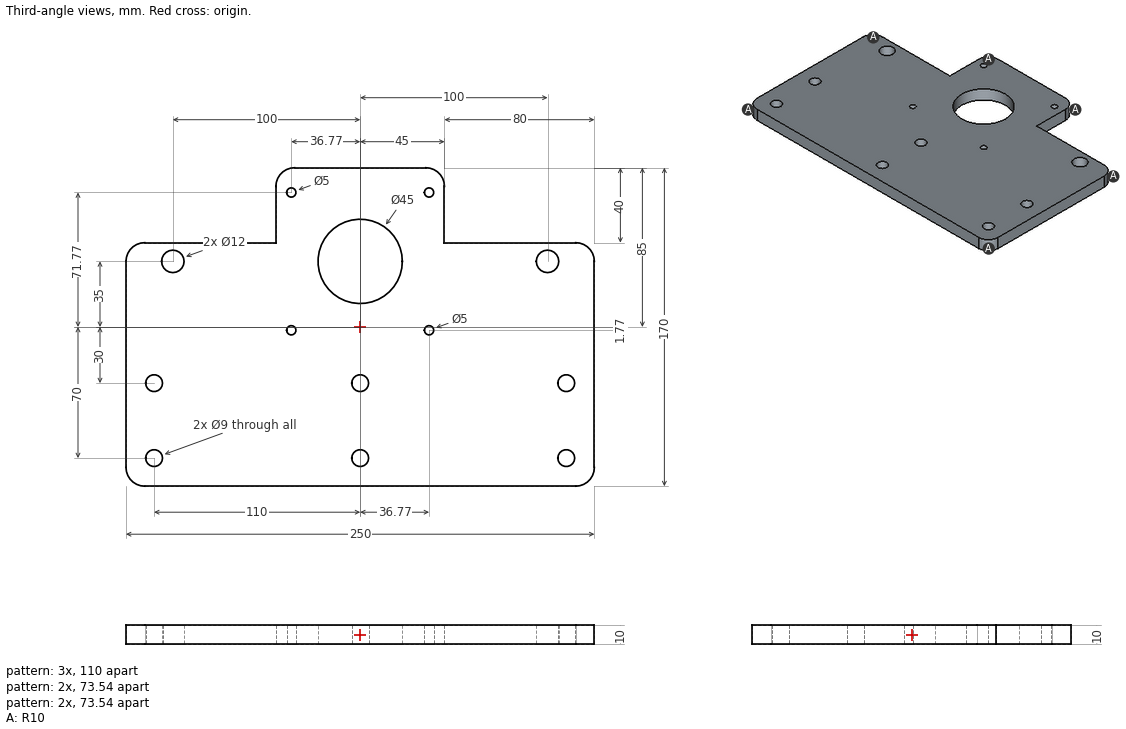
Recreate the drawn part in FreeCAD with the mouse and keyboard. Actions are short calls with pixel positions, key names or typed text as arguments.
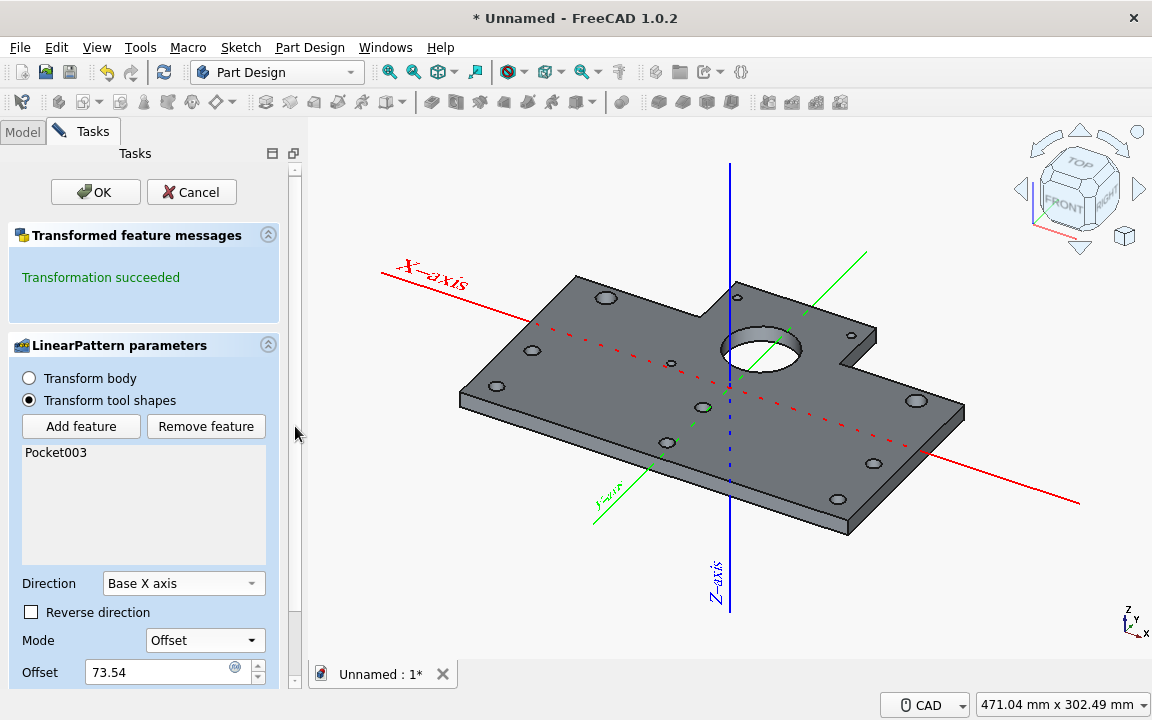
click(96, 192)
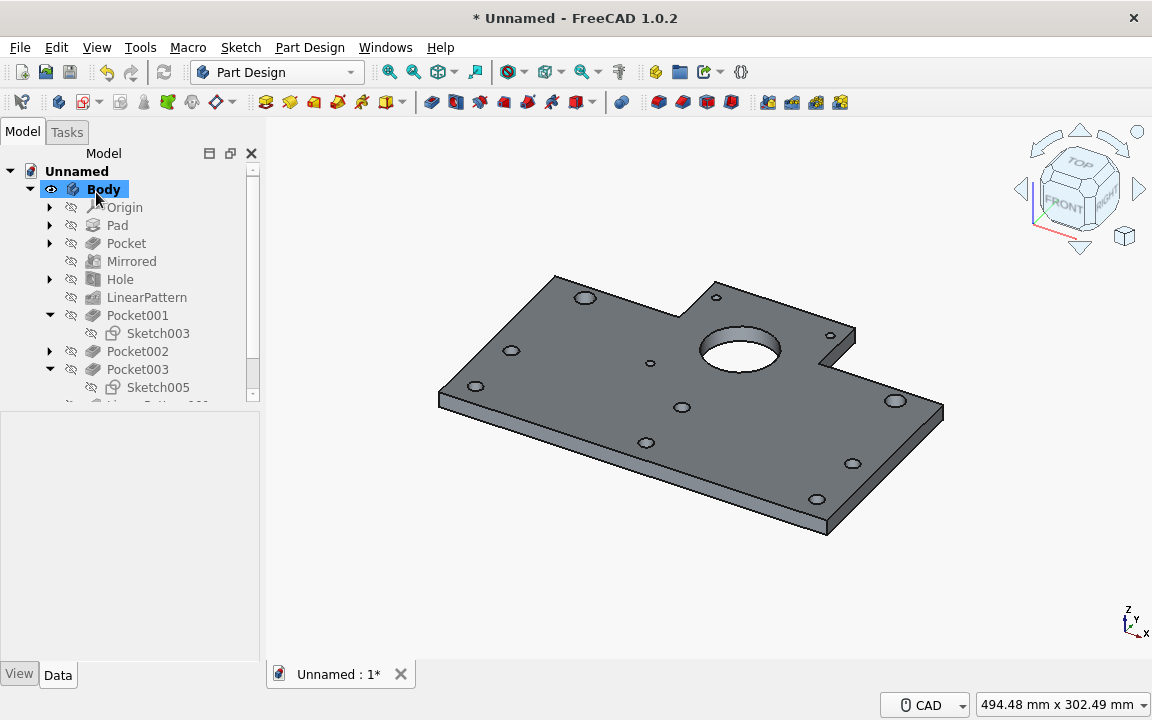
click(820, 416)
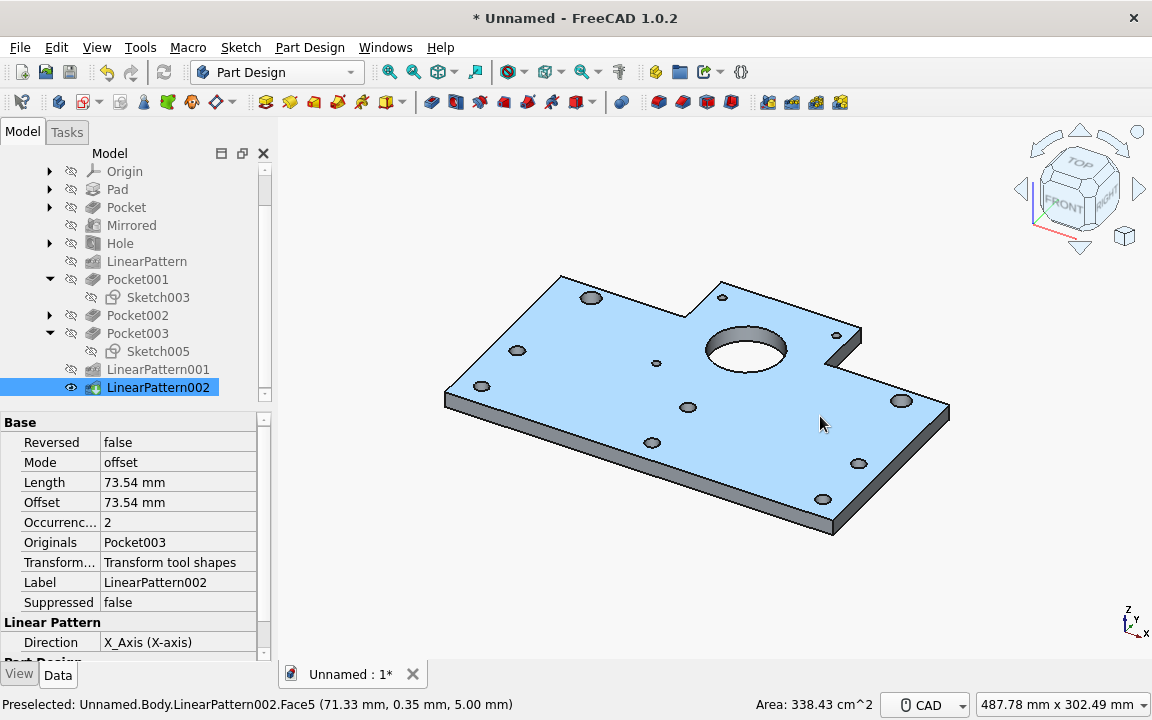
click(84, 102)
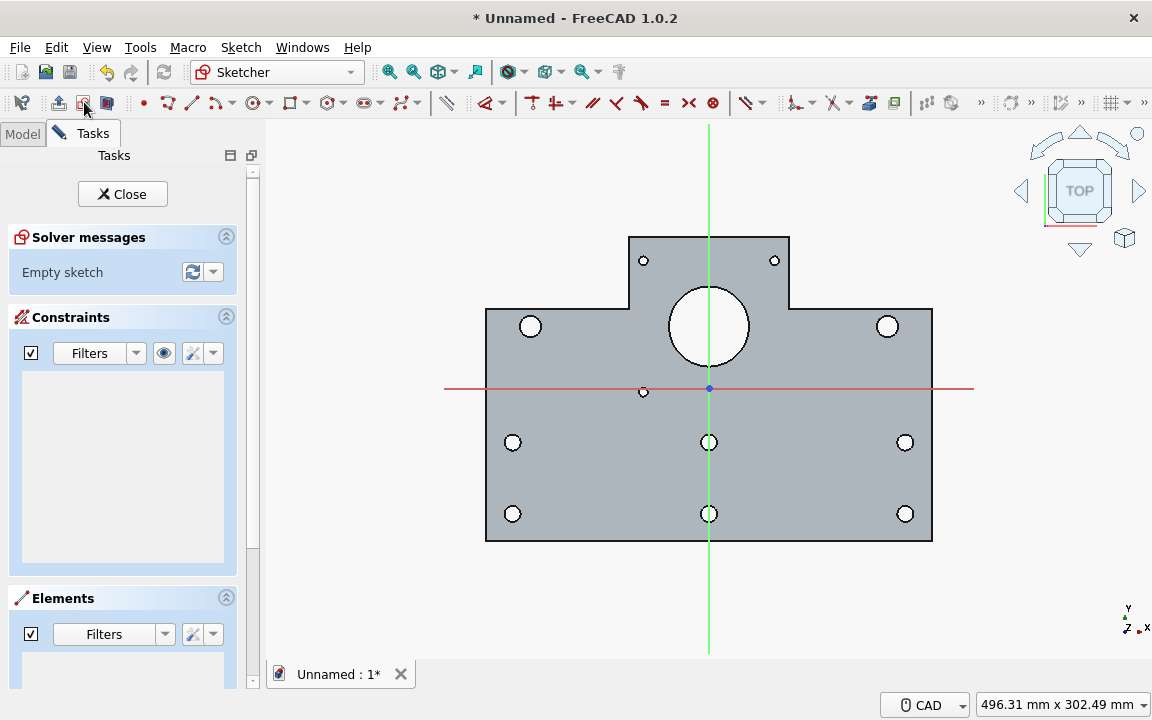
scroll(782, 392, up, 15)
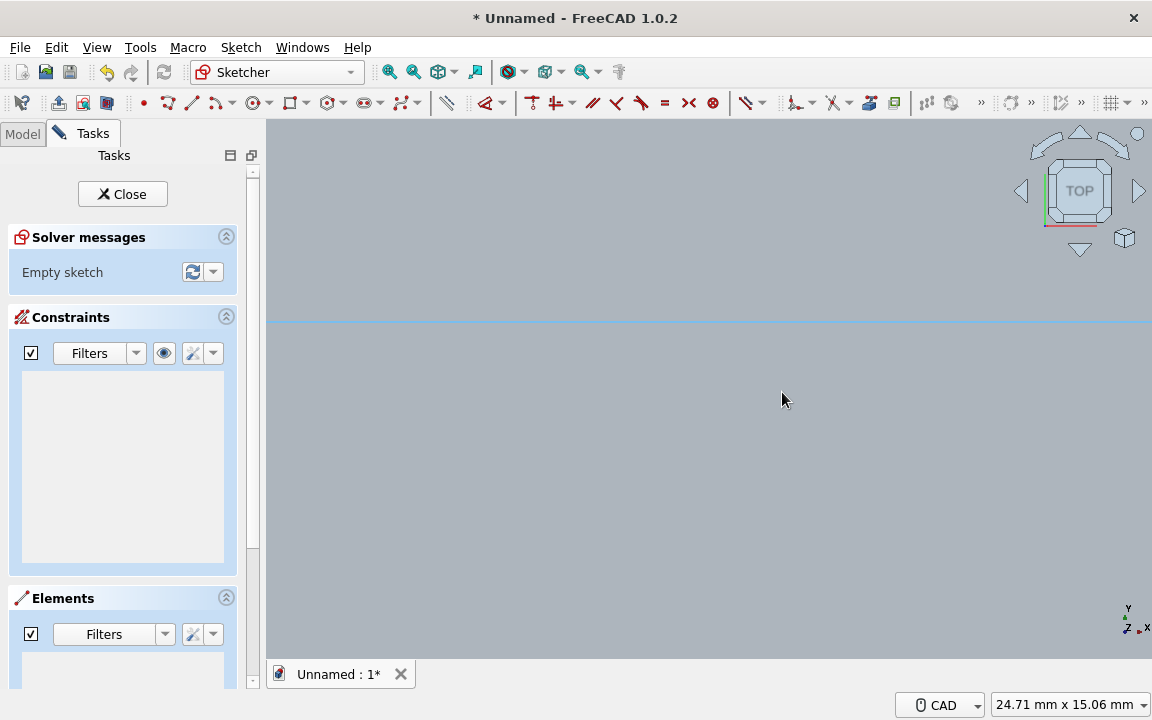
scroll(602, 381, up, 3)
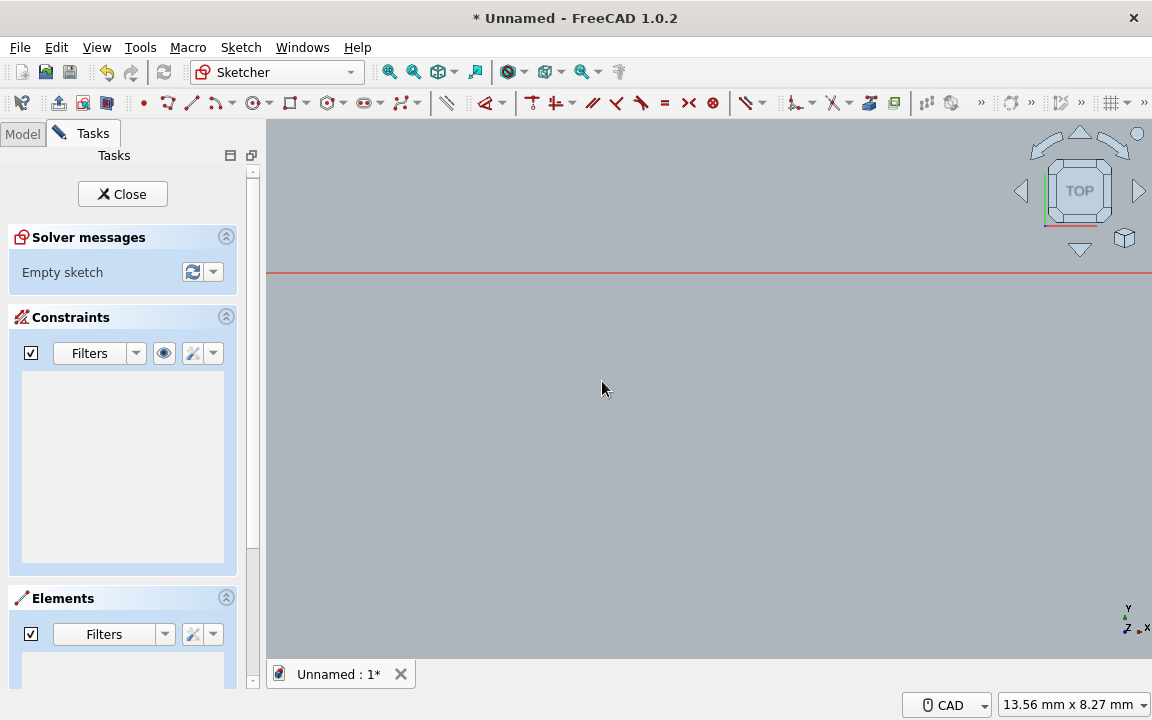
key(g)
key(c)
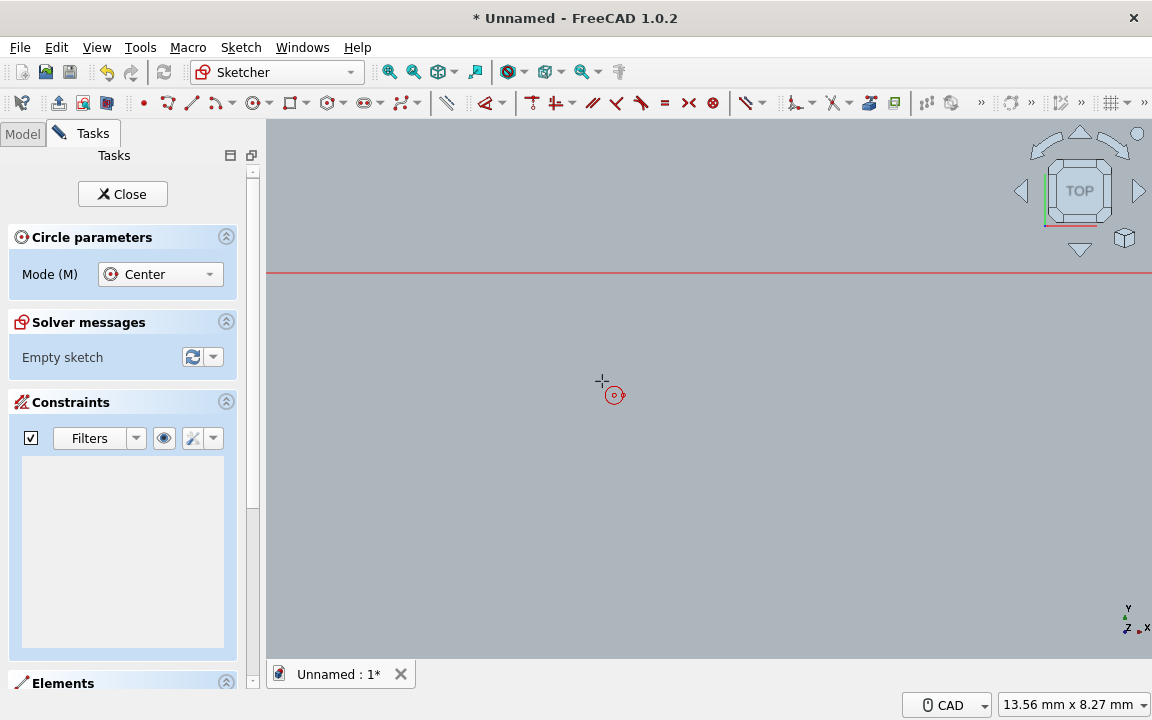
click(640, 389)
move(756, 504)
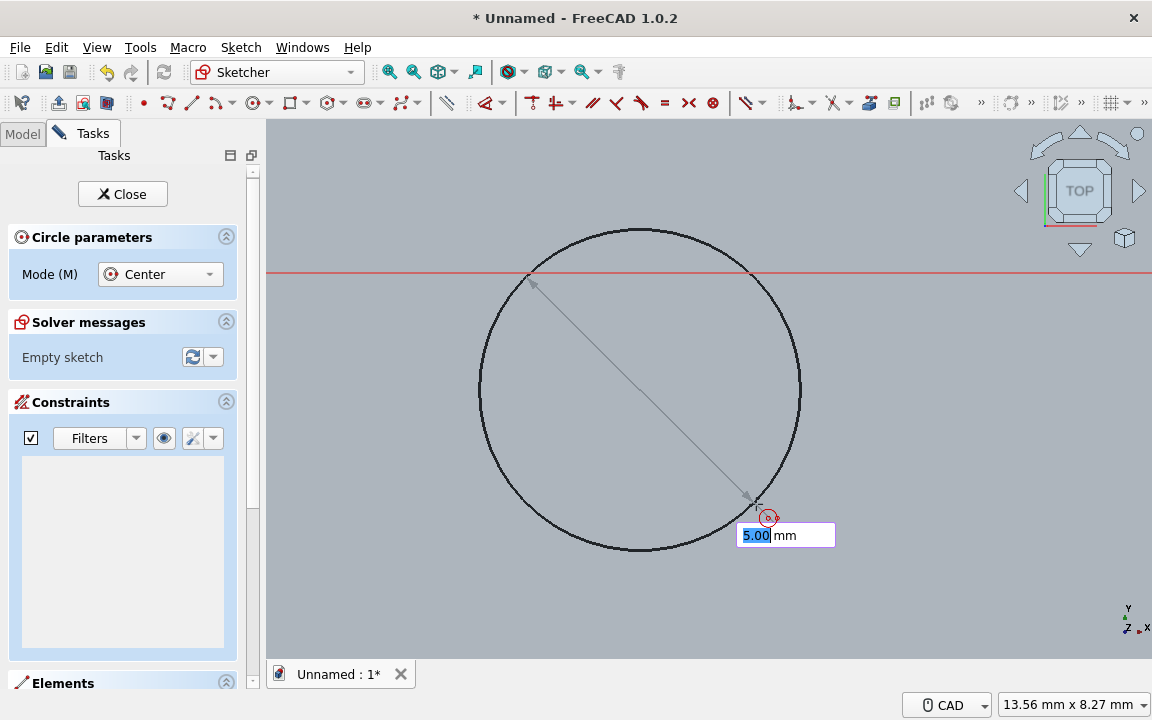
text(5)
key(Return)
key(Escape)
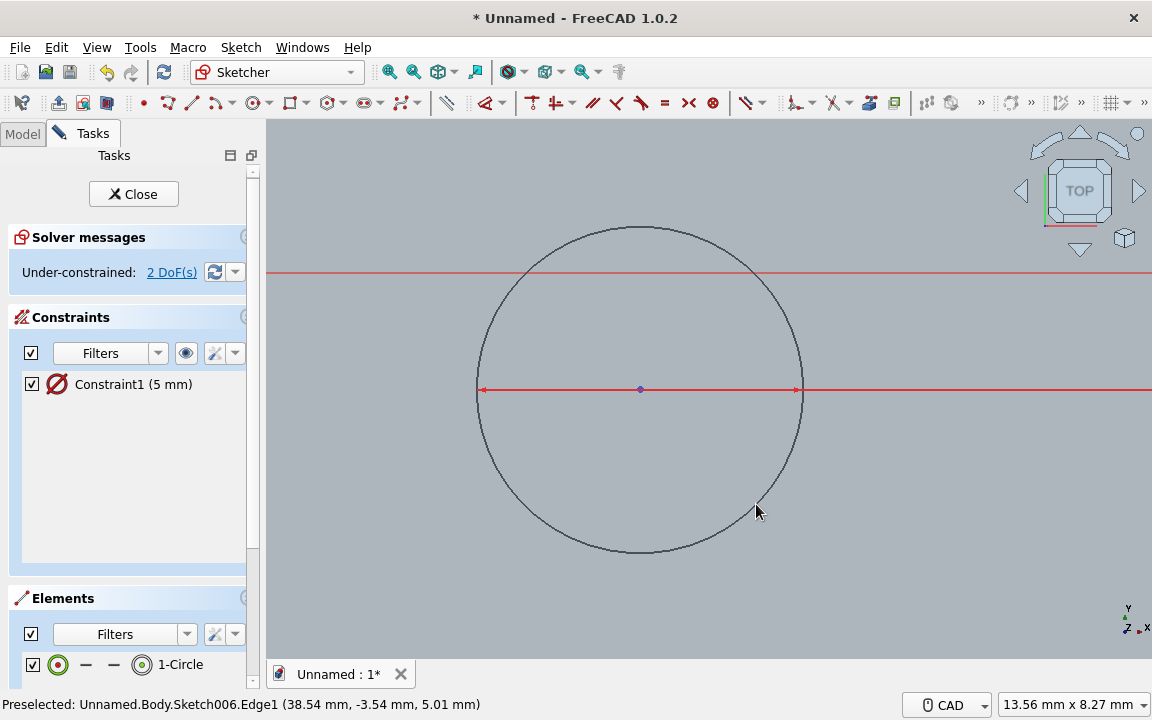
key(d)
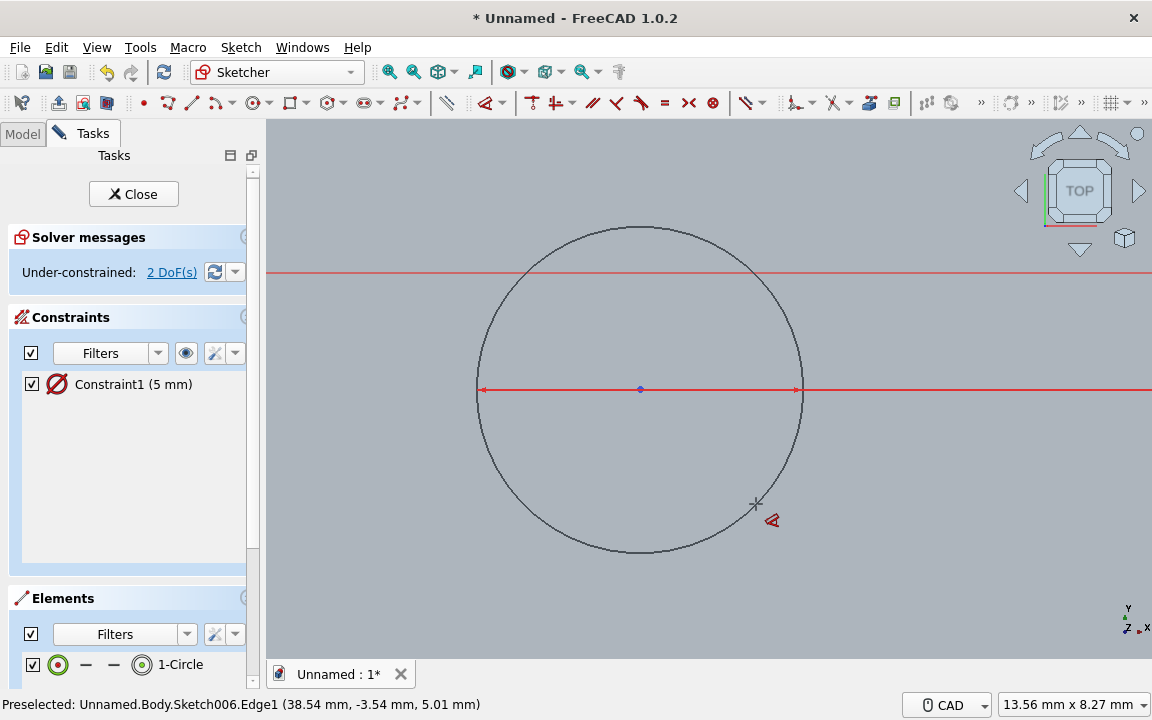
click(640, 390)
click(674, 332)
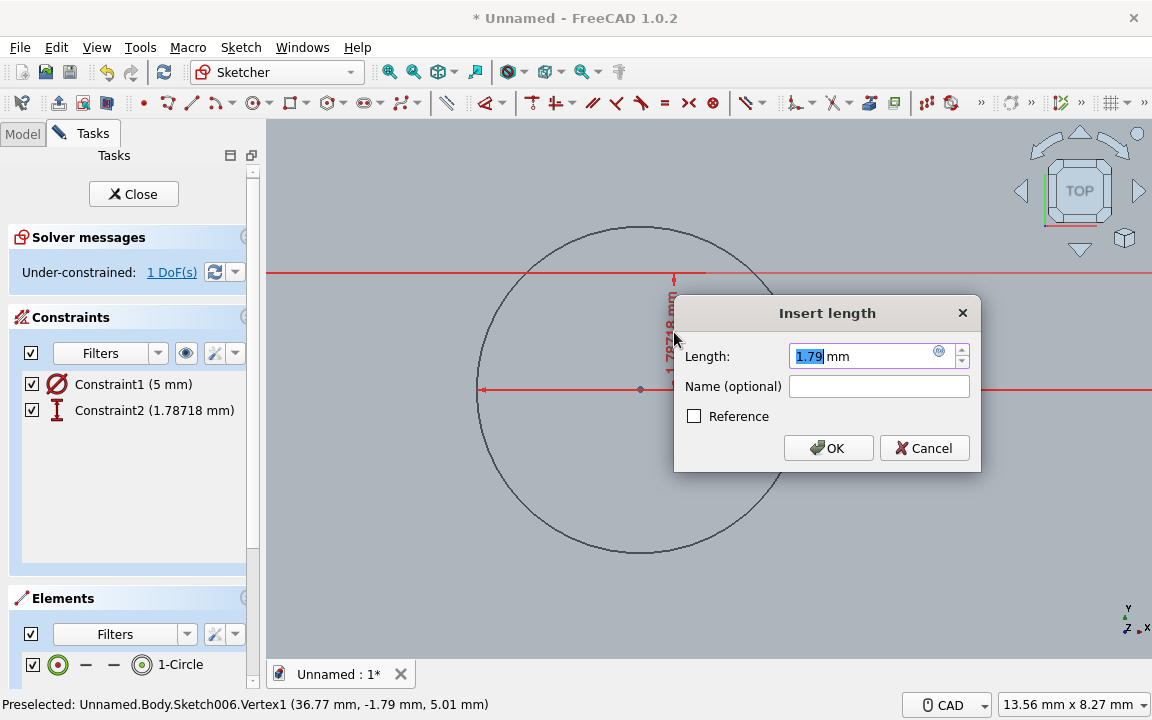
text(1.77)
key(Return)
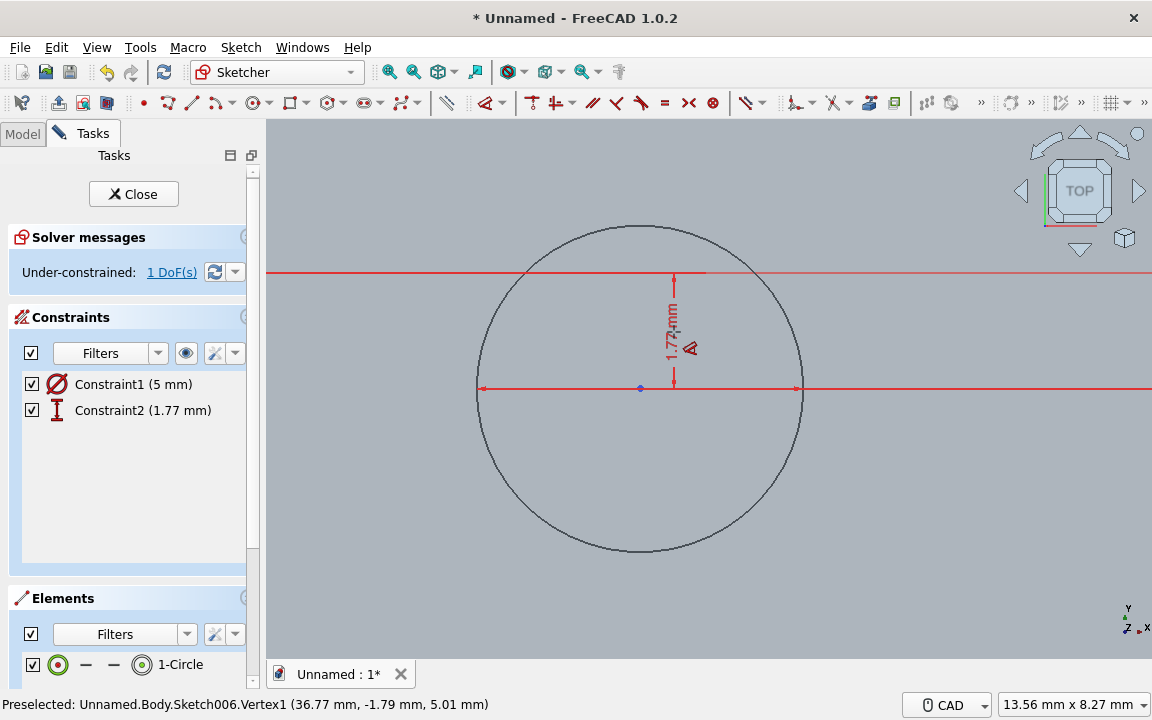
click(640, 389)
click(467, 239)